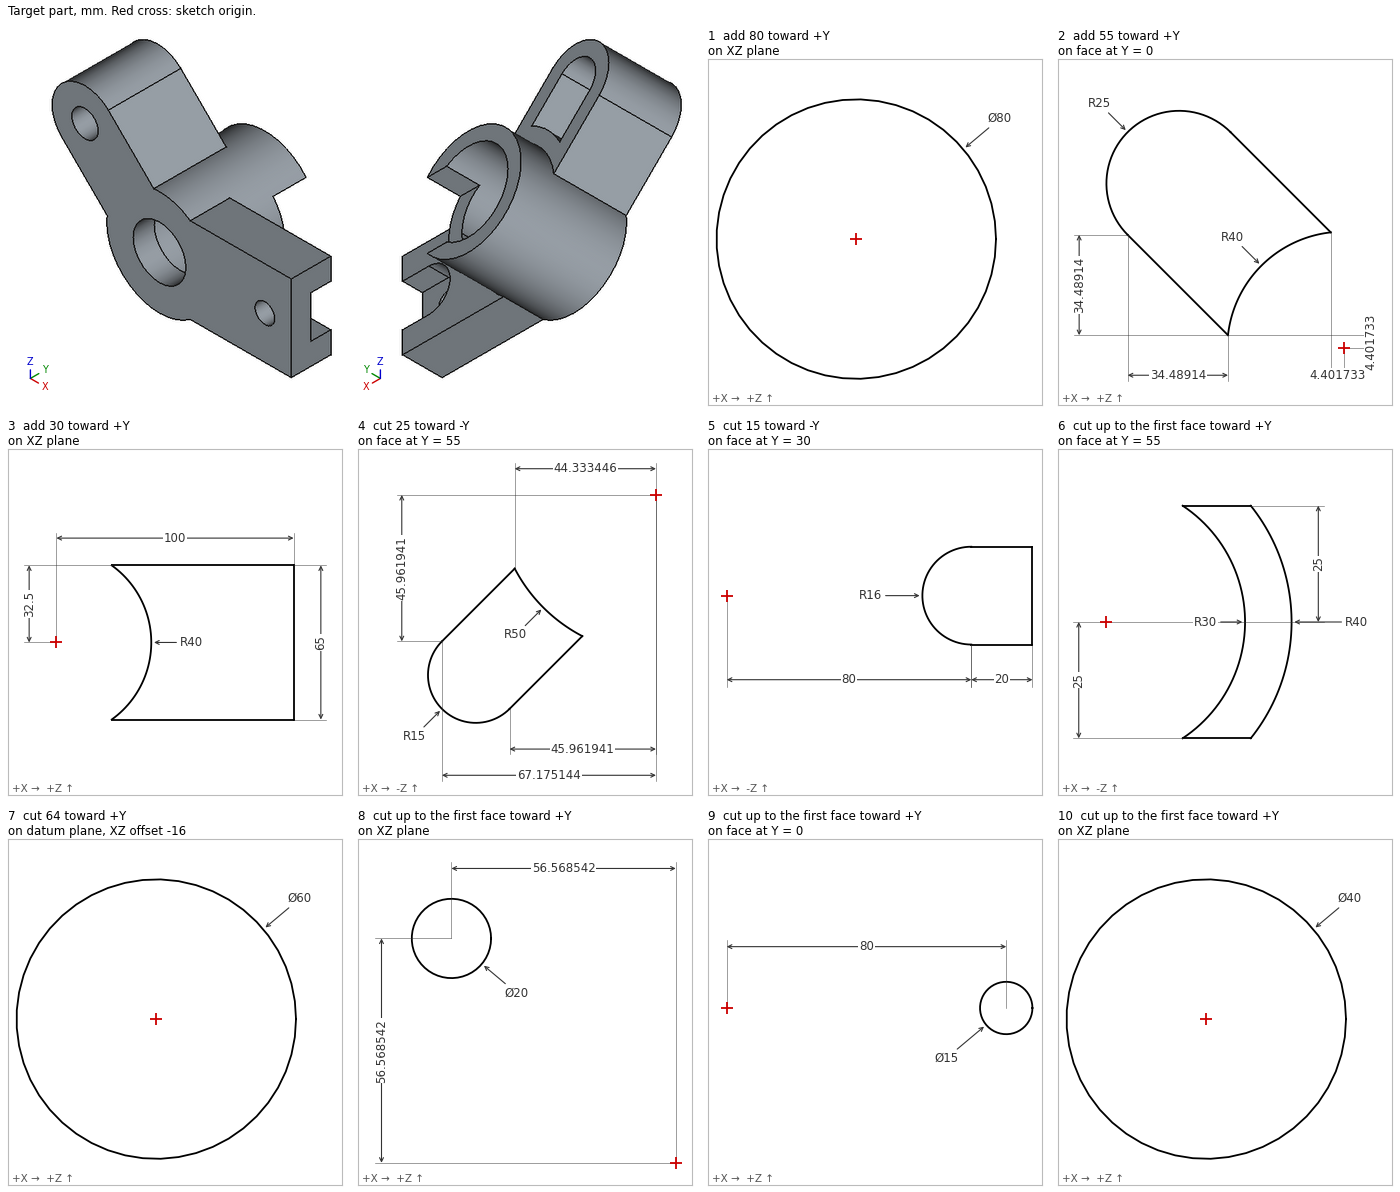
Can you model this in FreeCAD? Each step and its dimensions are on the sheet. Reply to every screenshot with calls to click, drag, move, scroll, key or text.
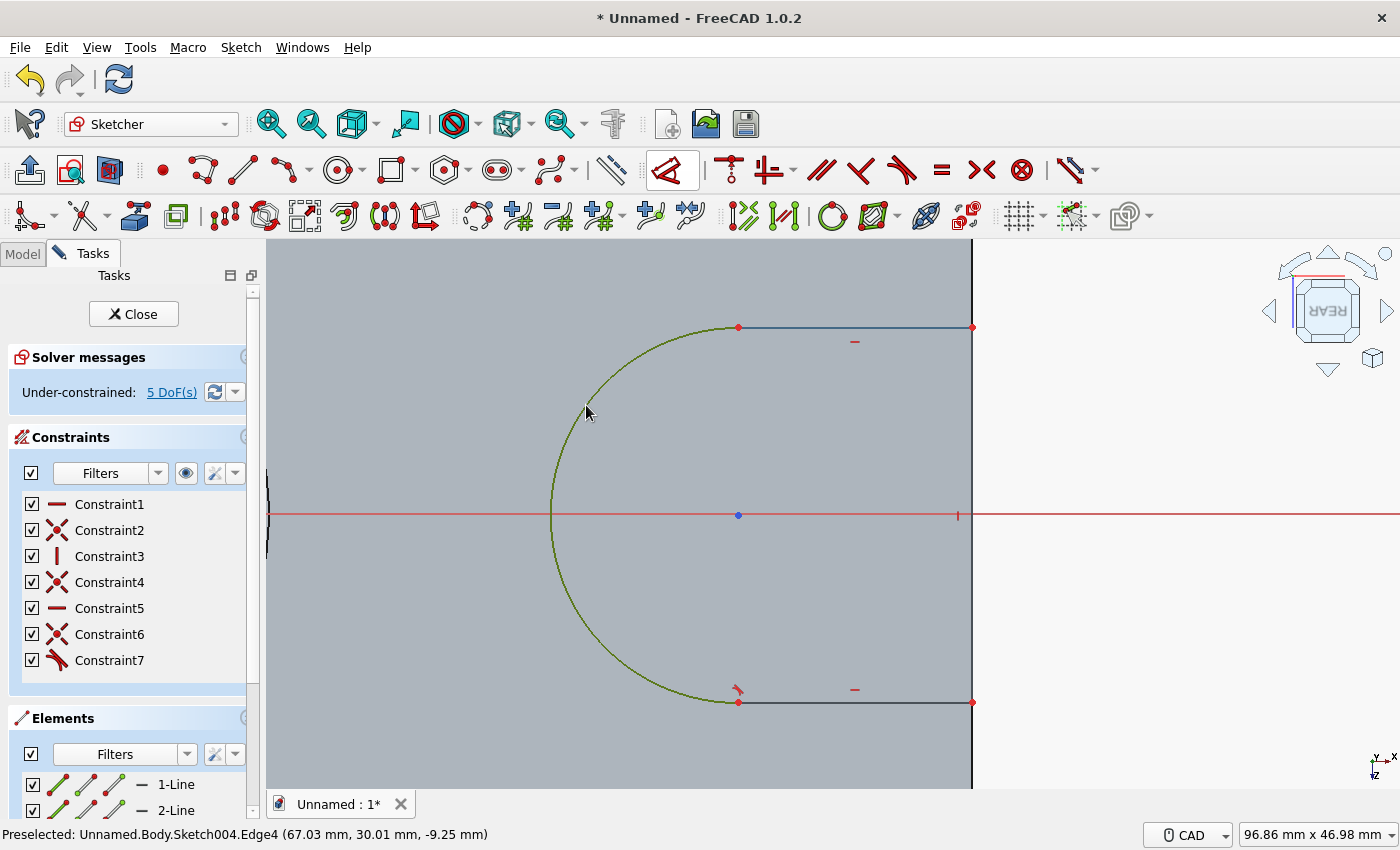
click(902, 170)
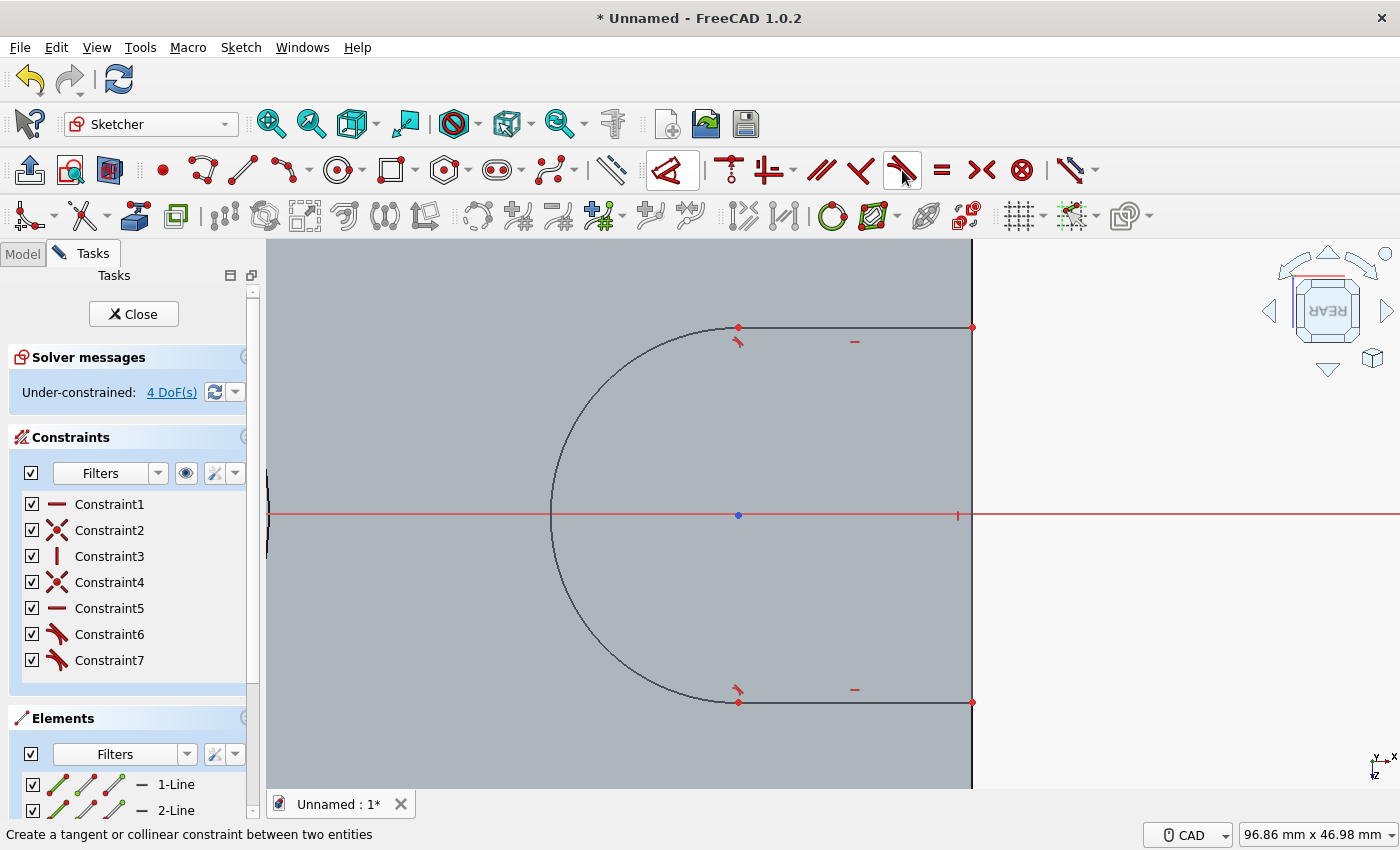
click(738, 516)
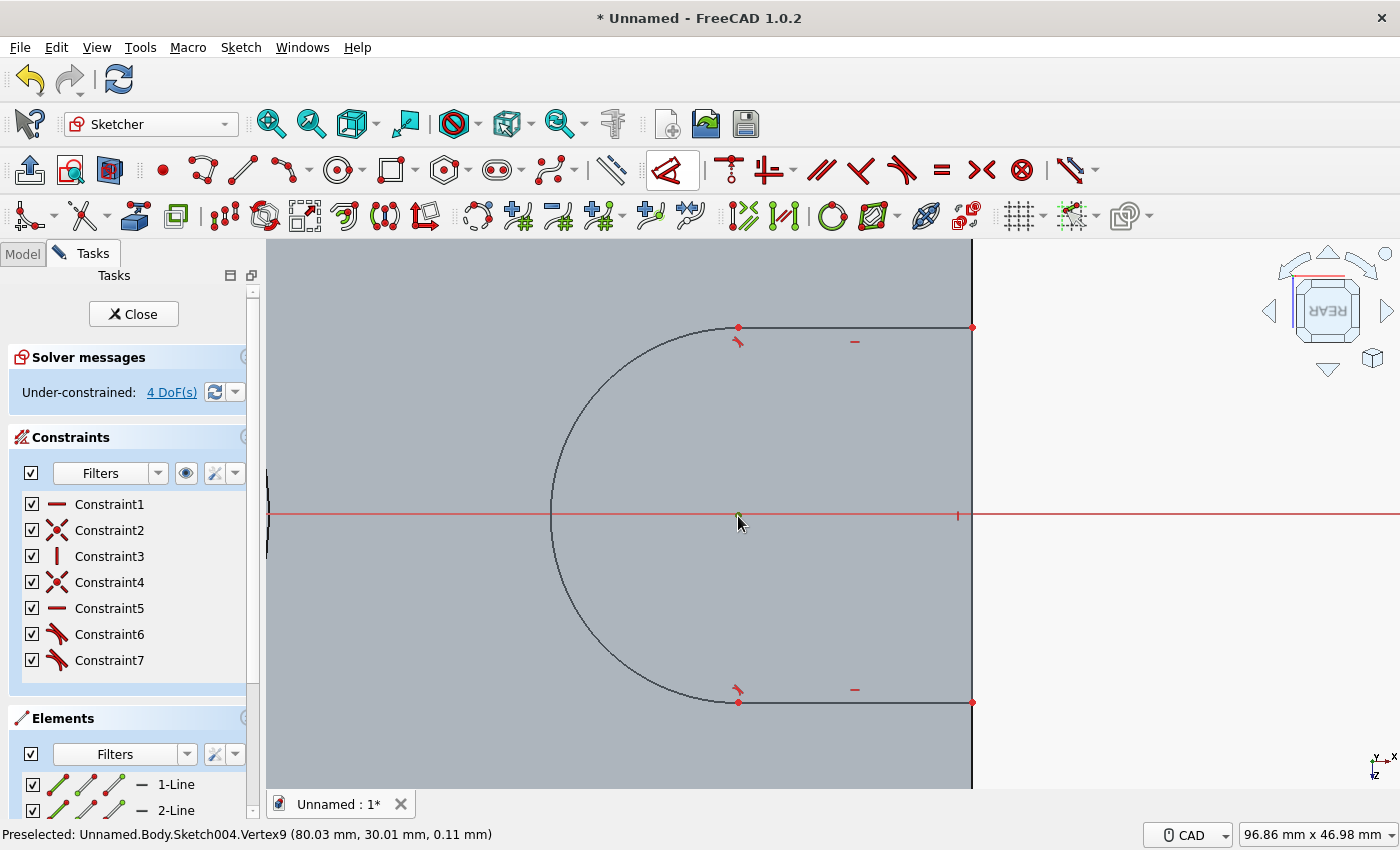
click(361, 514)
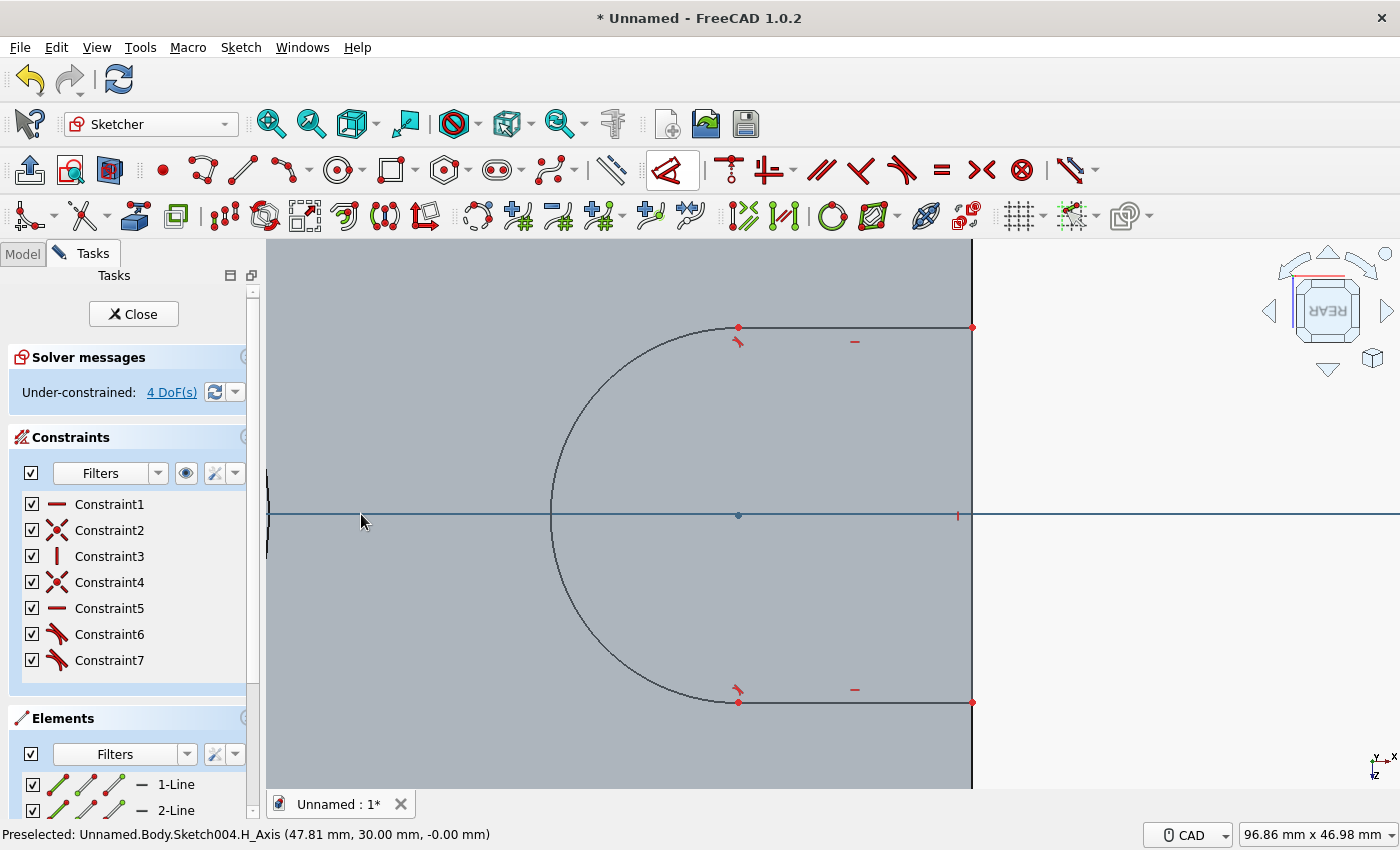
click(730, 170)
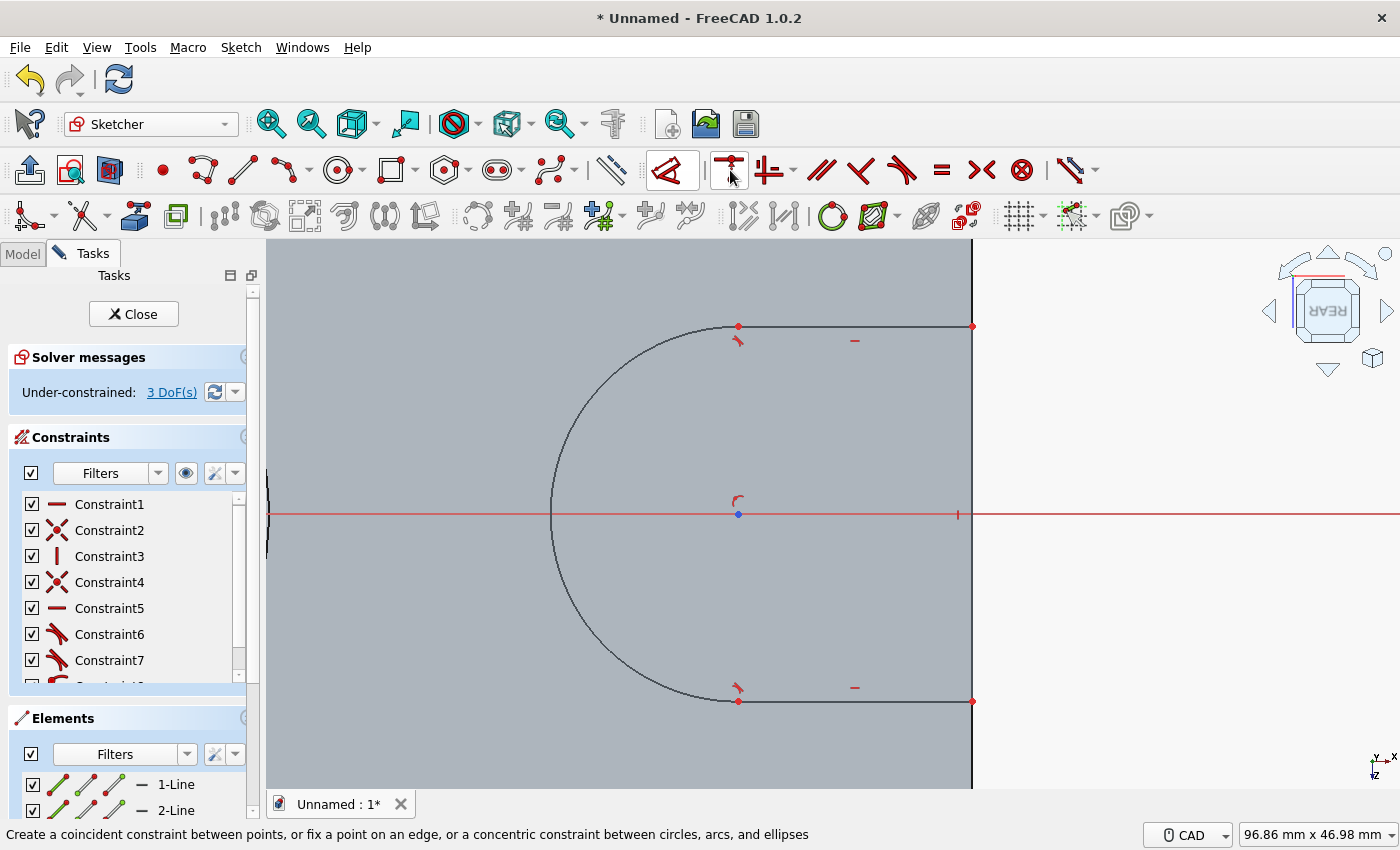
click(586, 404)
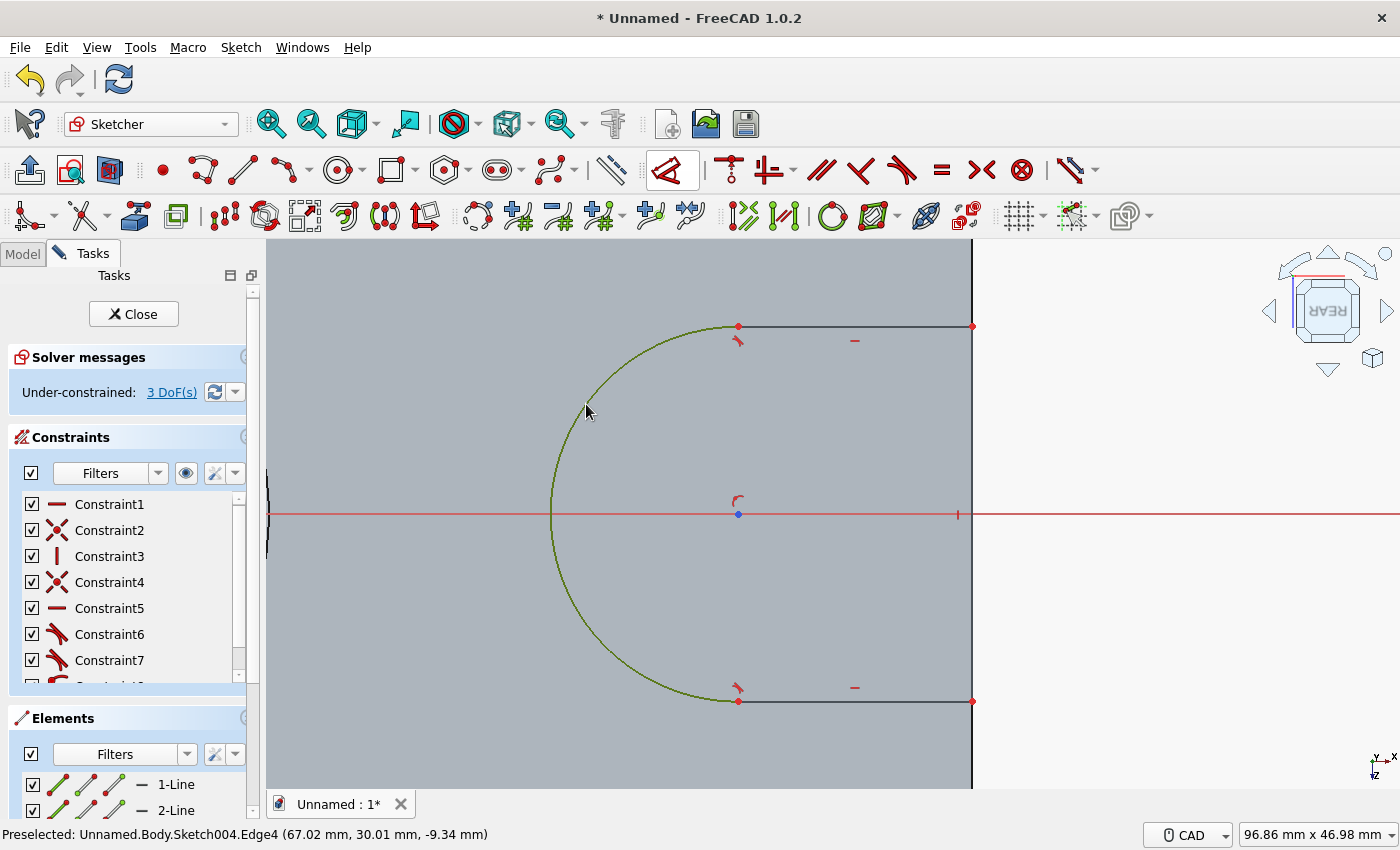
click(694, 170)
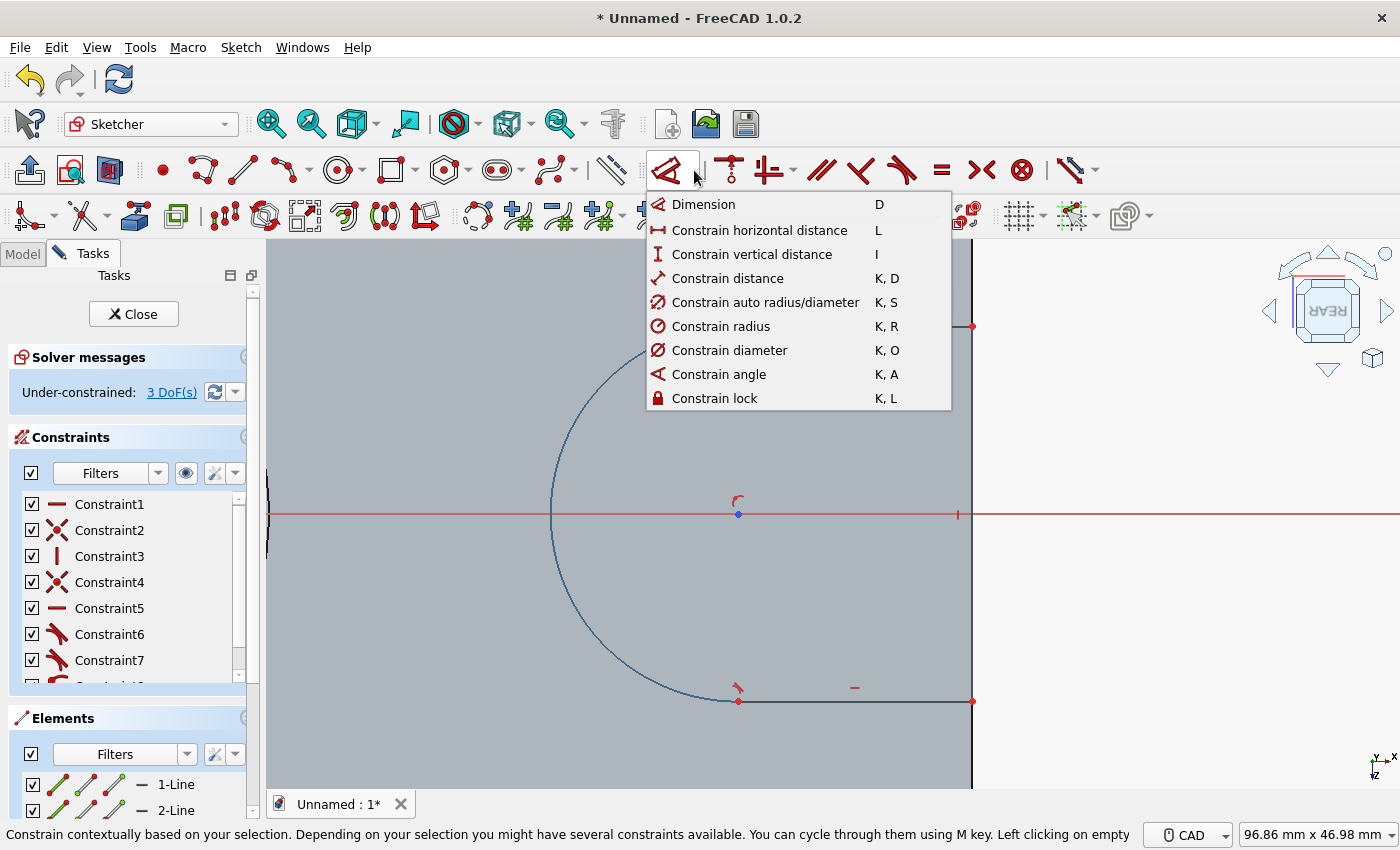
click(799, 326)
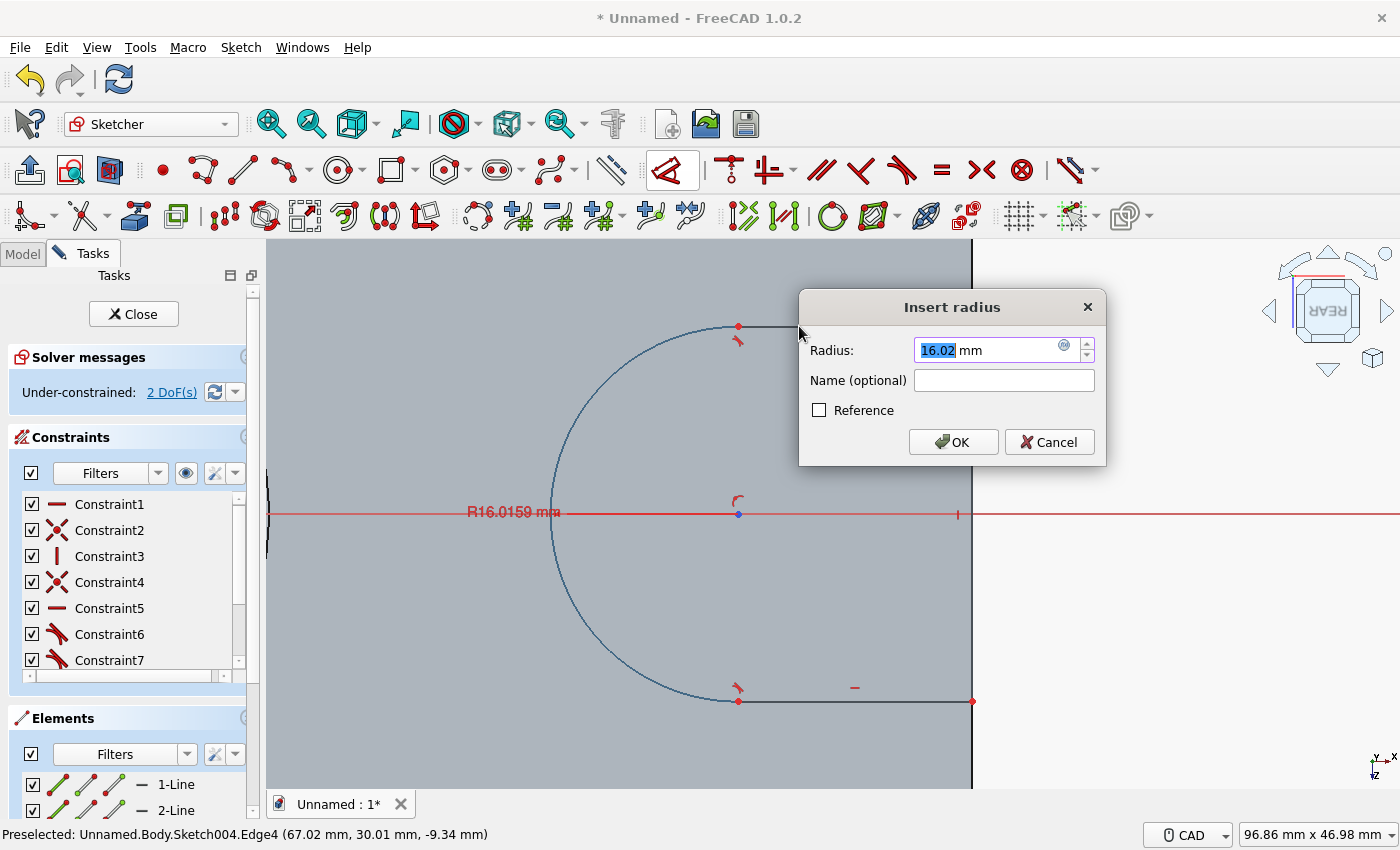
text(16)
key(Return)